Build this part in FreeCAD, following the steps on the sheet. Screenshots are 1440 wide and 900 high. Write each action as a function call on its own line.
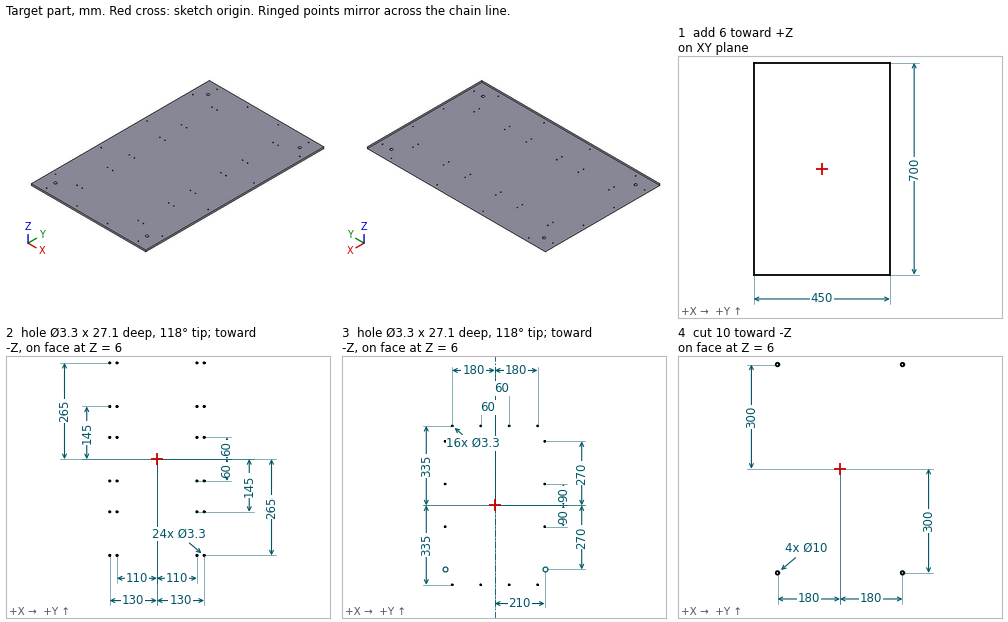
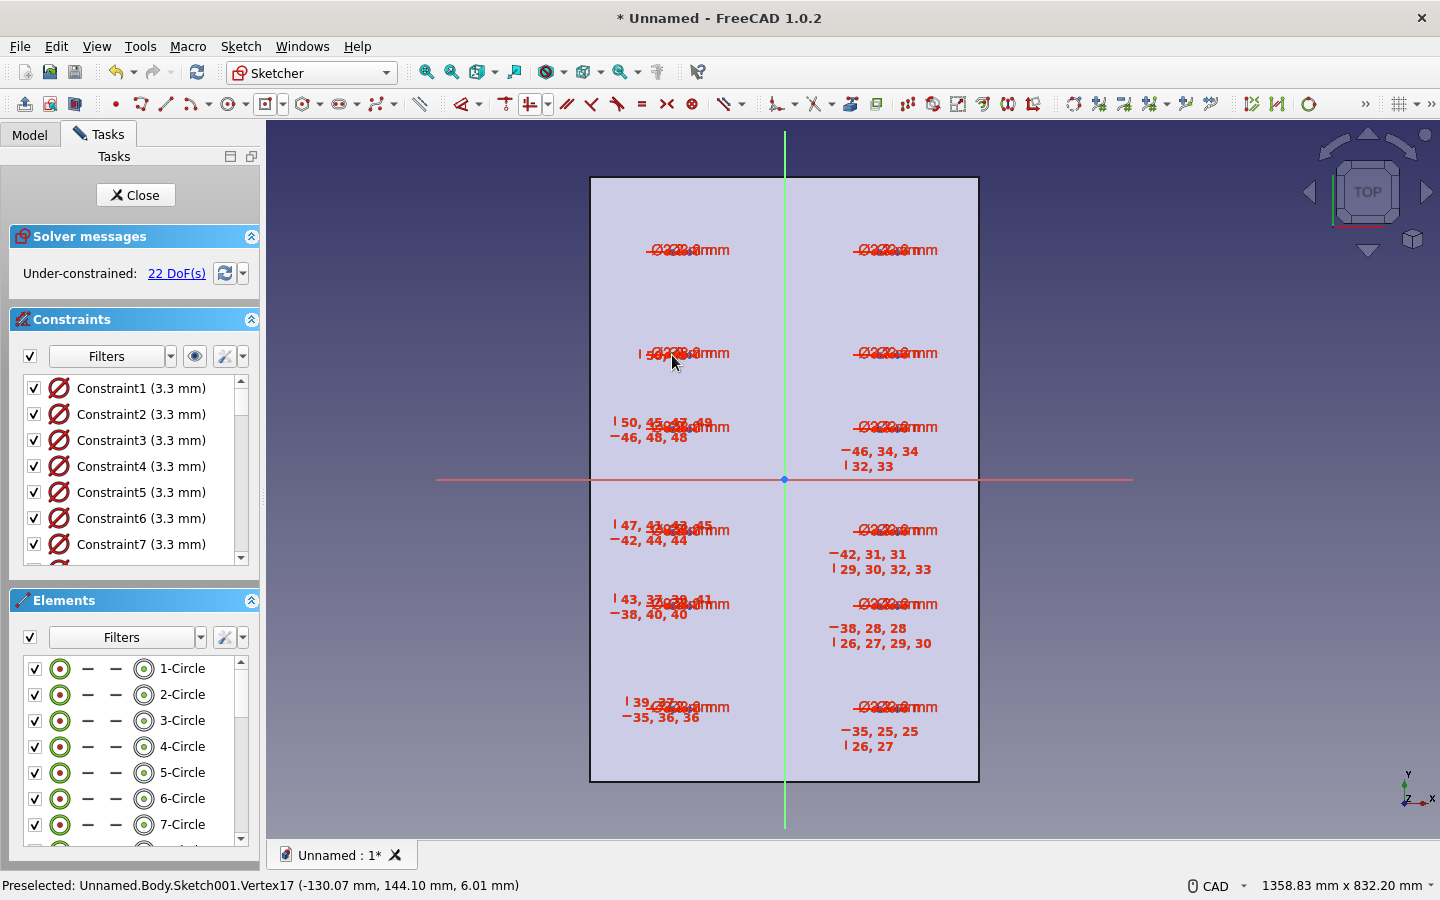
click(689, 355)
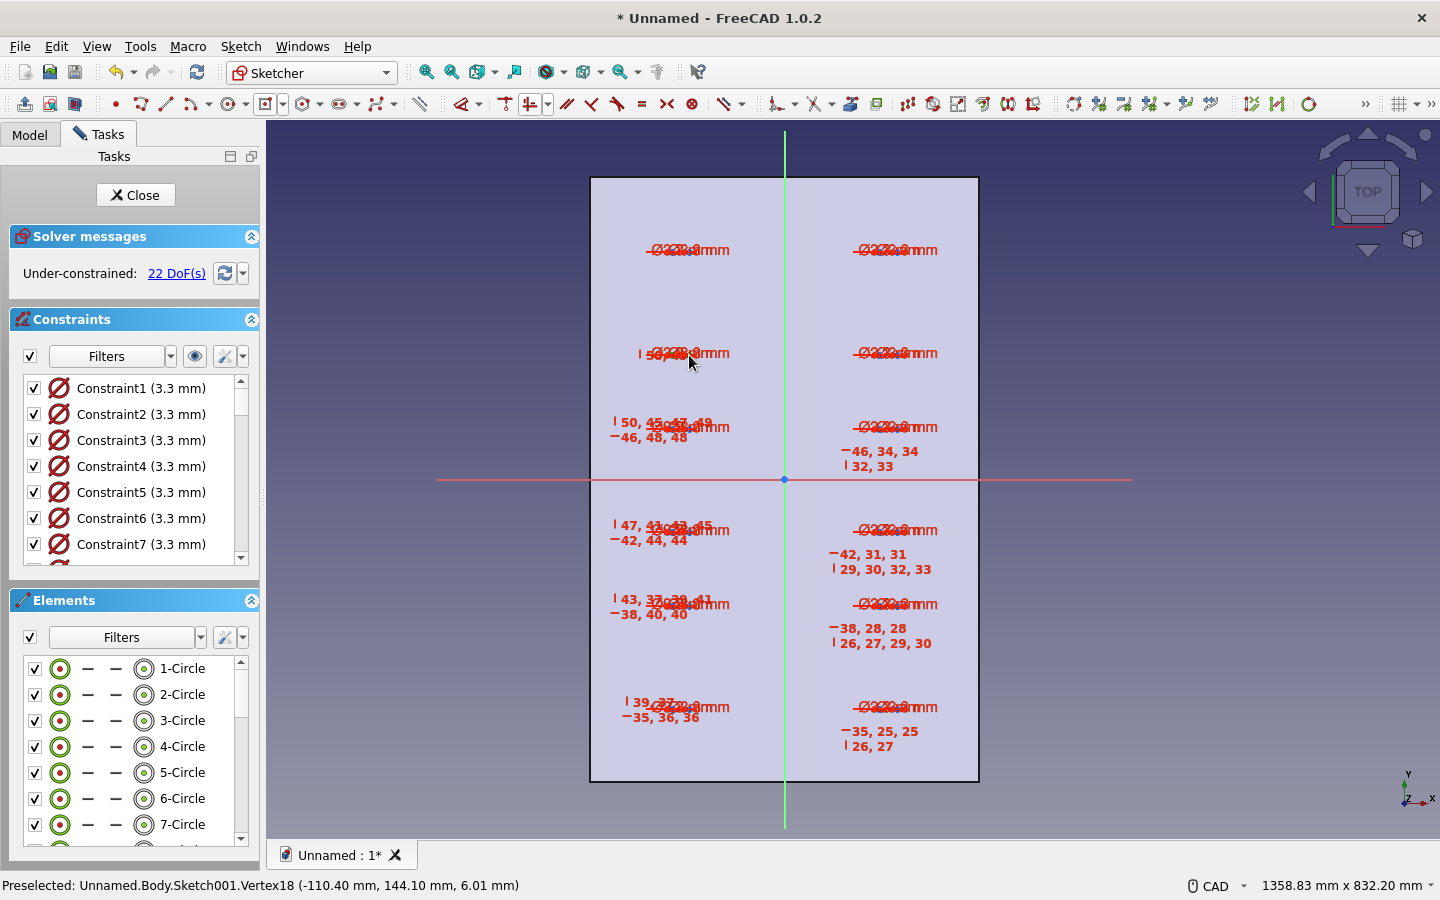
click(548, 104)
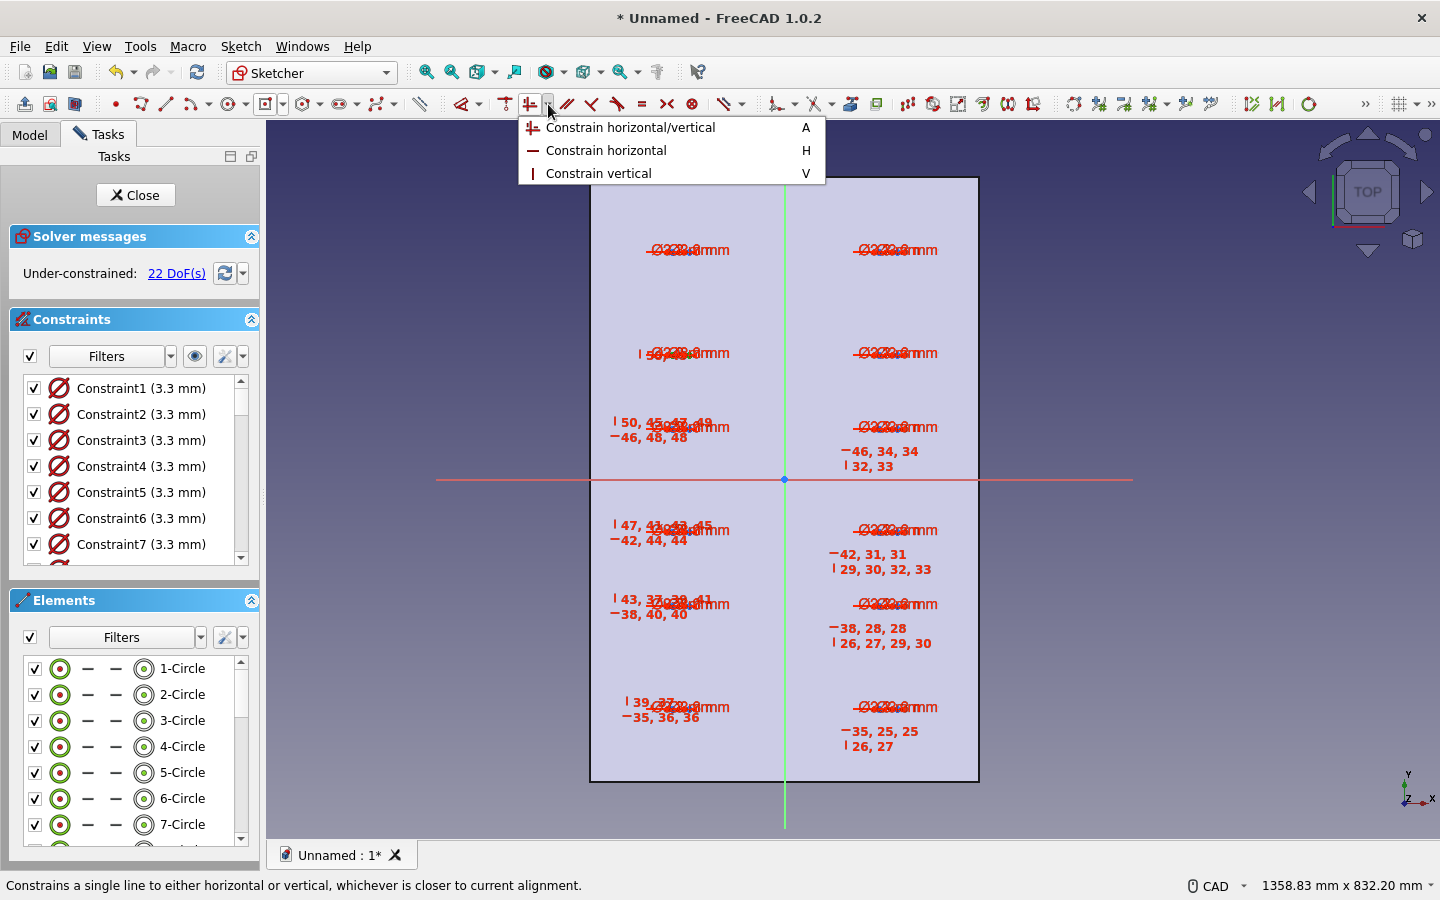
click(672, 150)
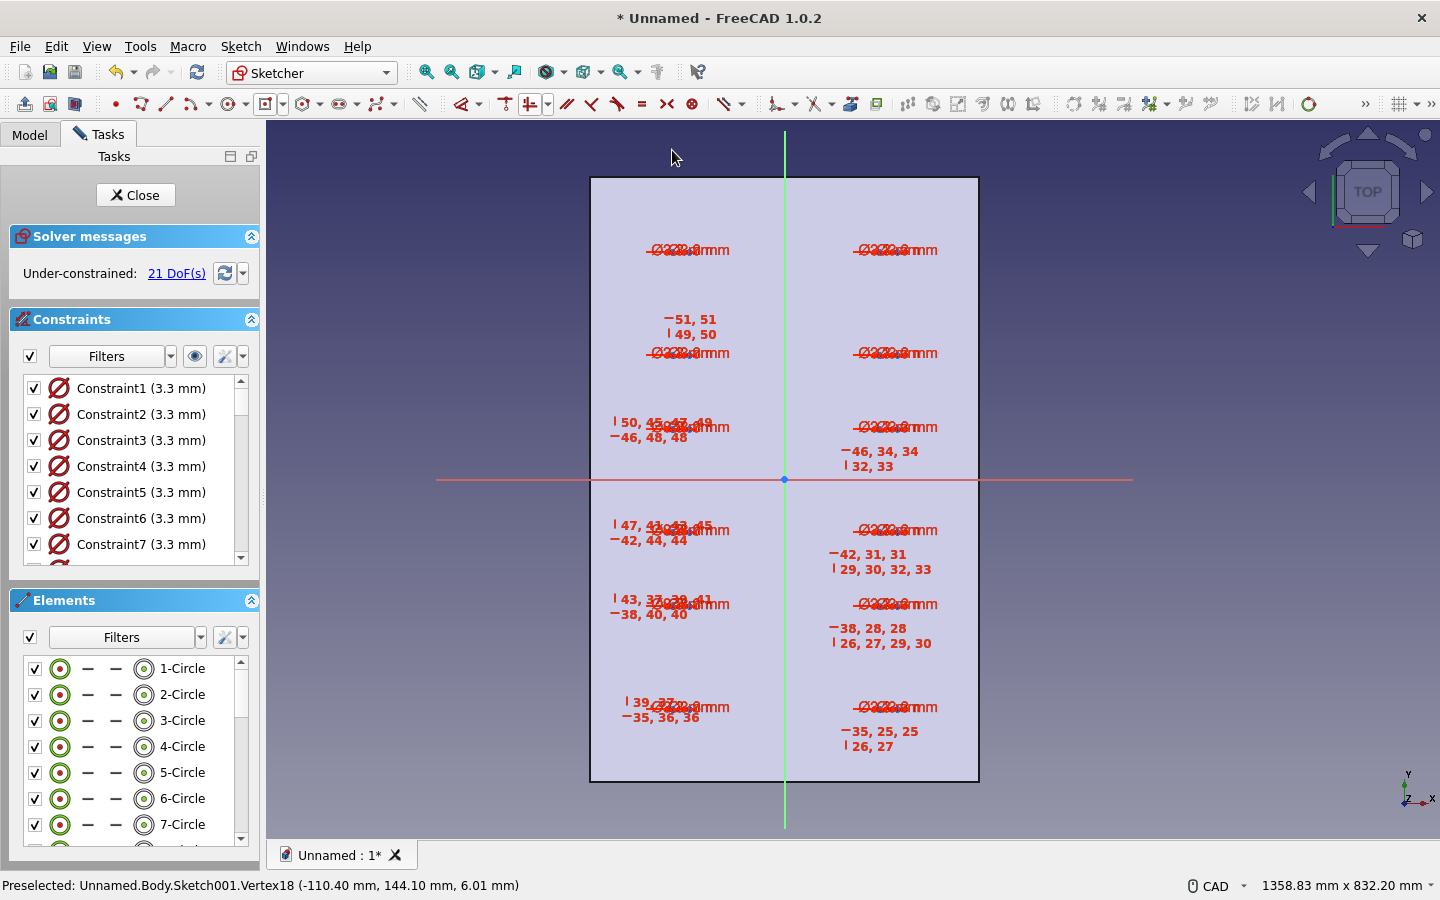
click(672, 355)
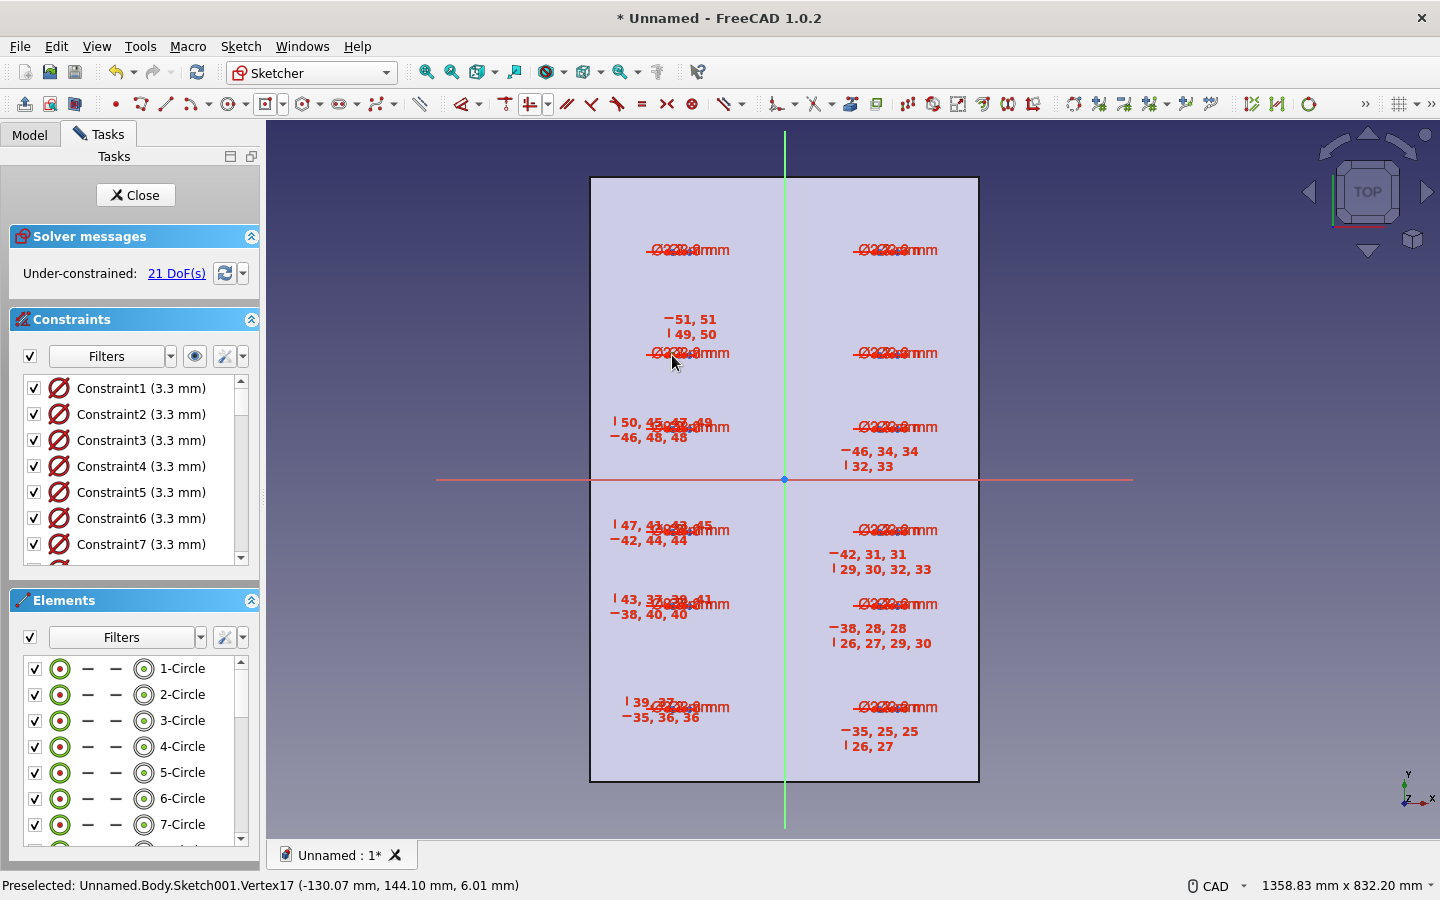
click(672, 252)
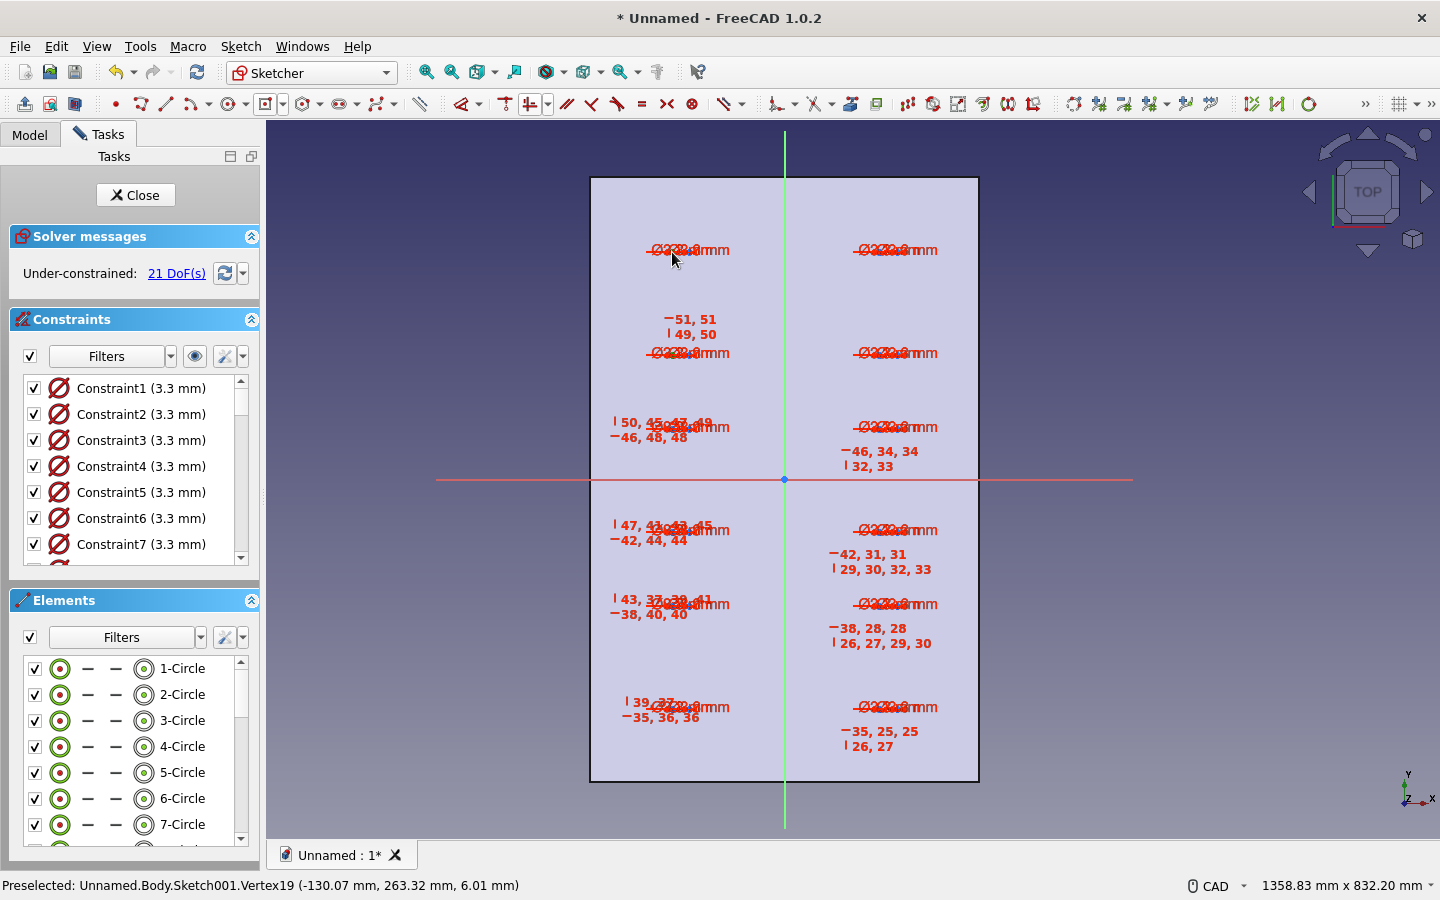
key(v)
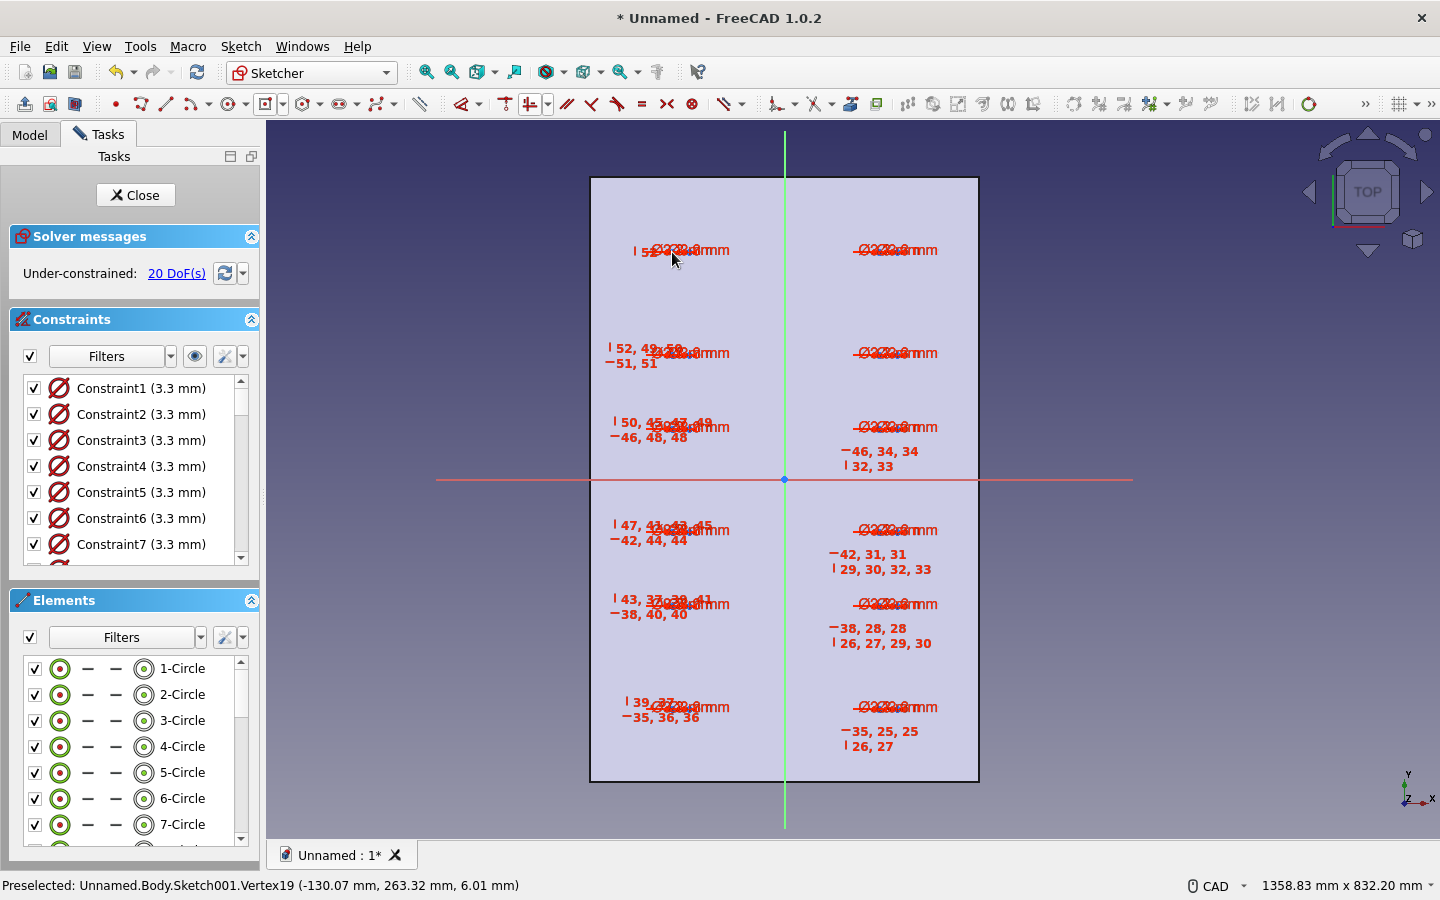
click(689, 355)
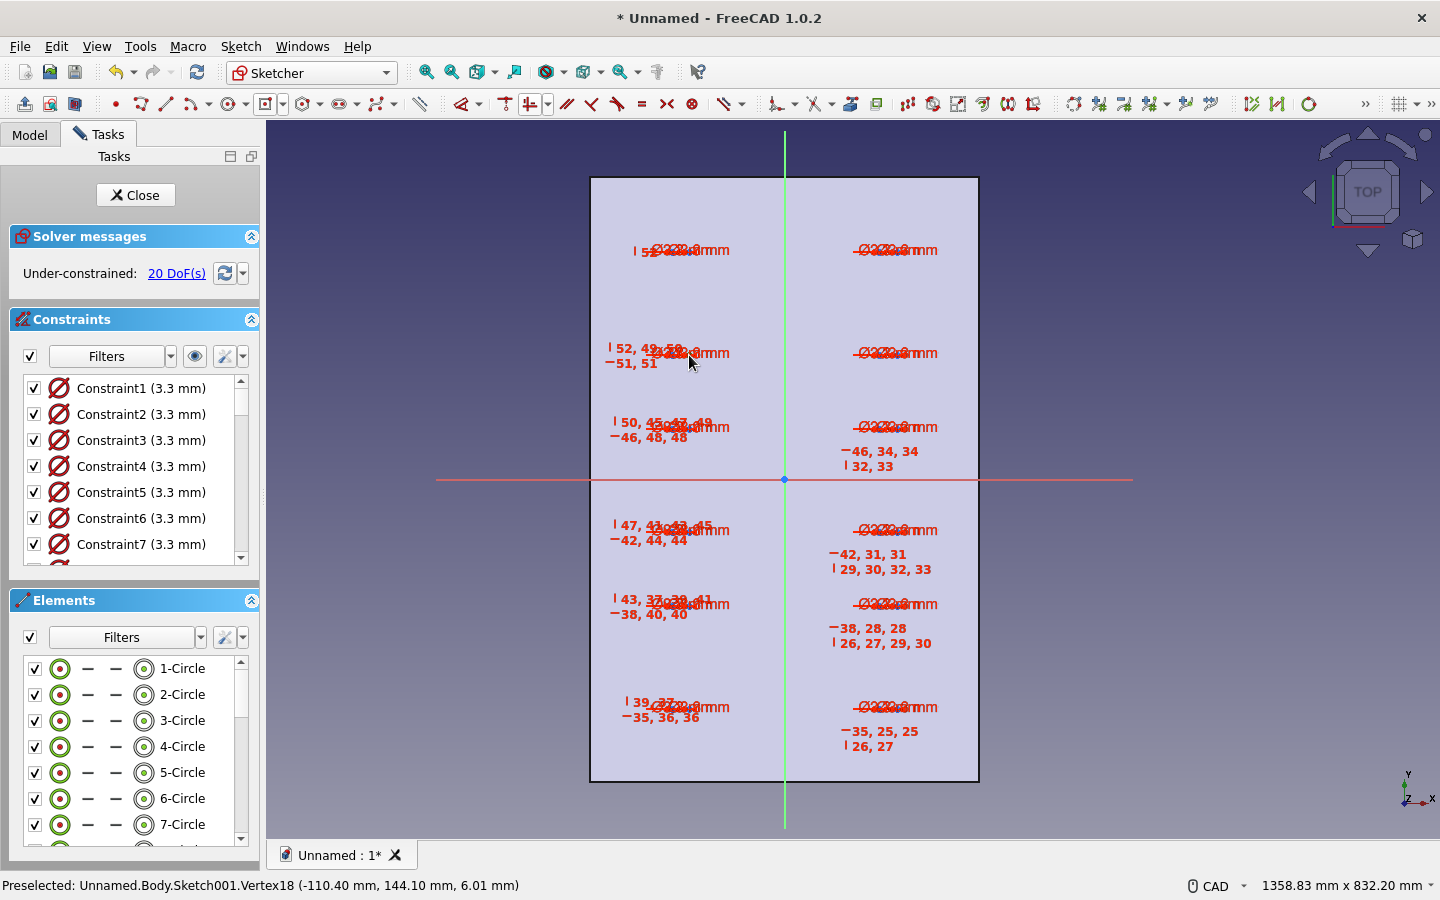
click(689, 252)